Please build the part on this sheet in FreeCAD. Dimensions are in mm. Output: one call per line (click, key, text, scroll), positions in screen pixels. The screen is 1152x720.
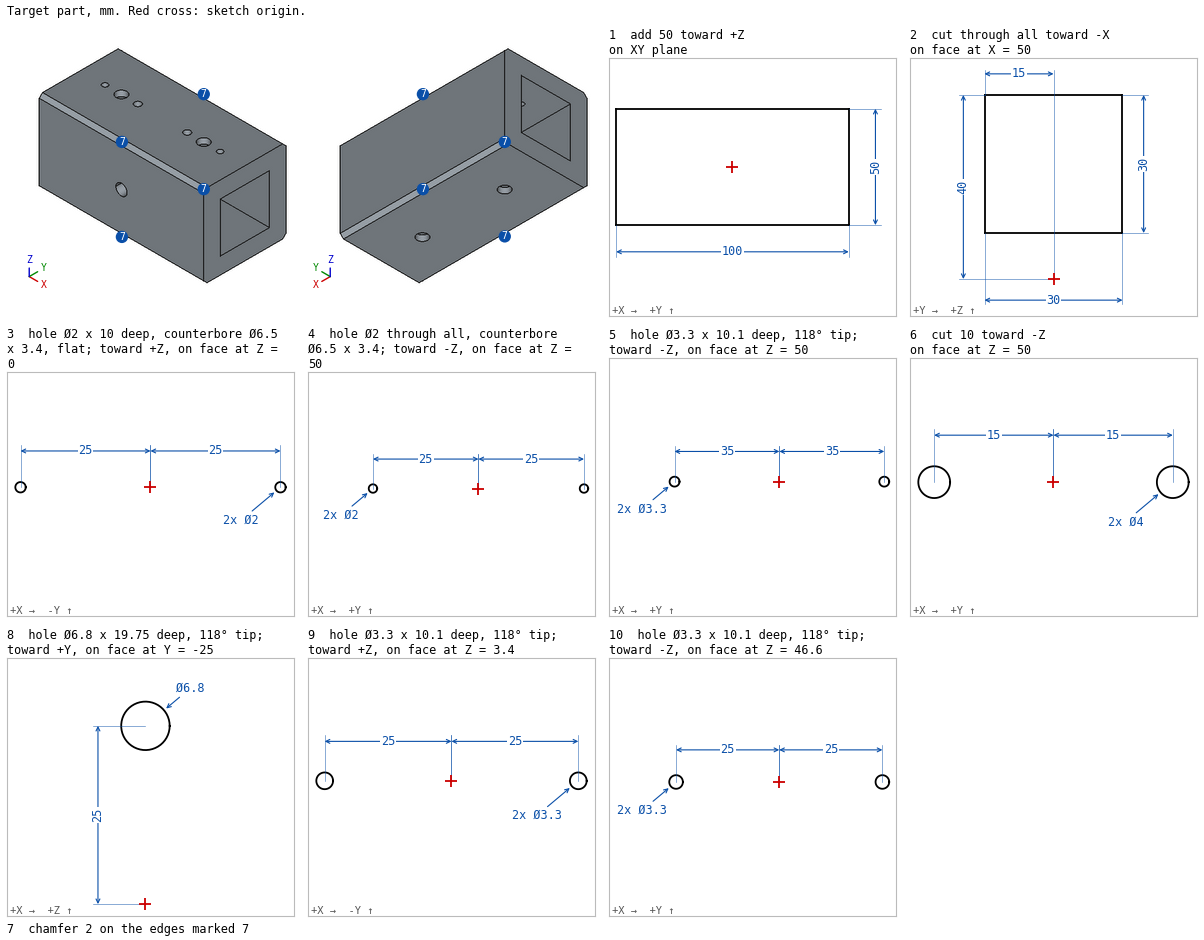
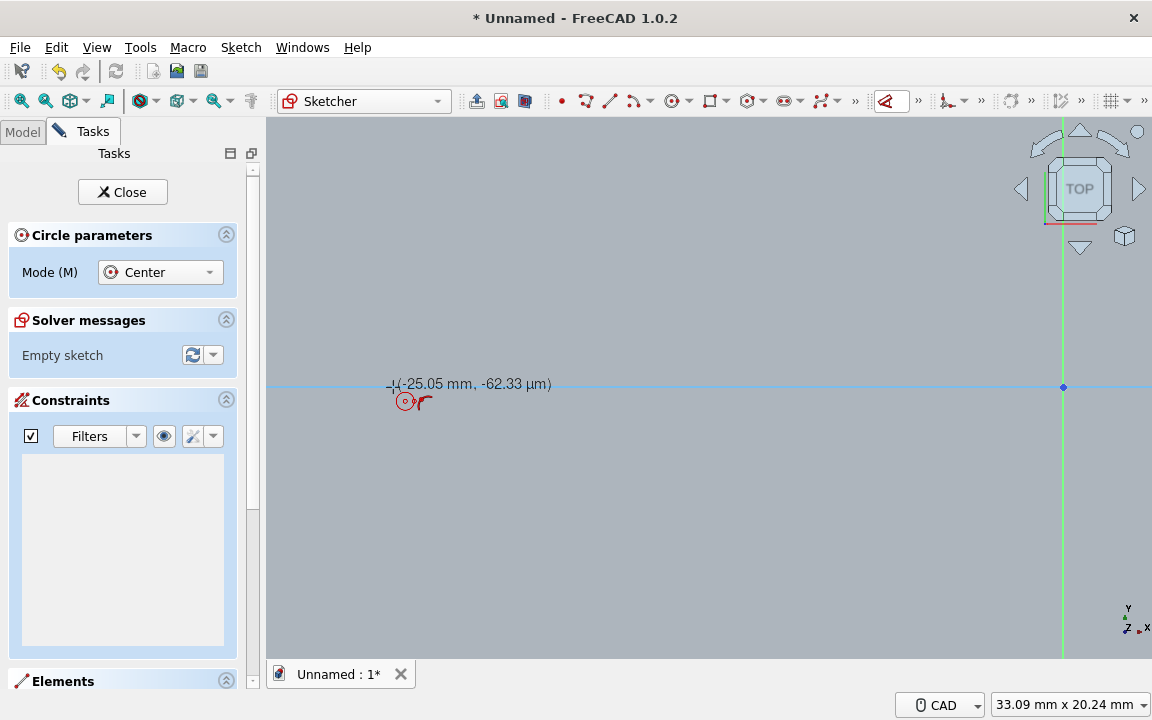
click(394, 387)
move(413, 368)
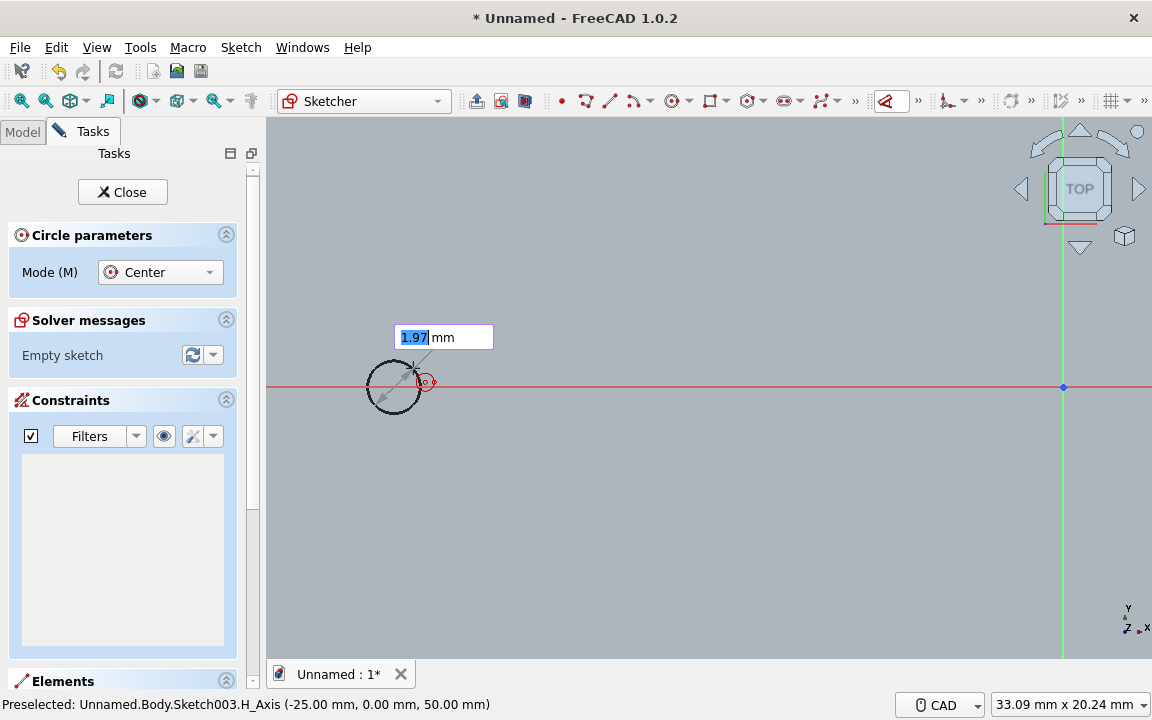
text(2)
key(Return)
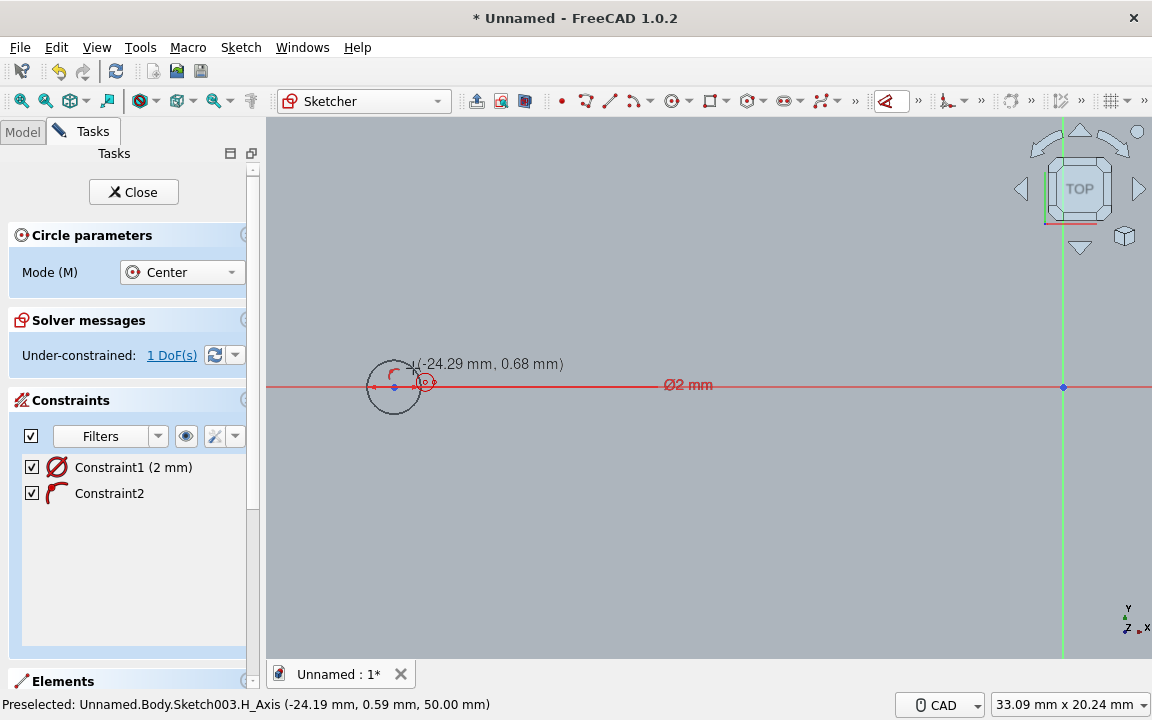
scroll(394, 388, down, 5)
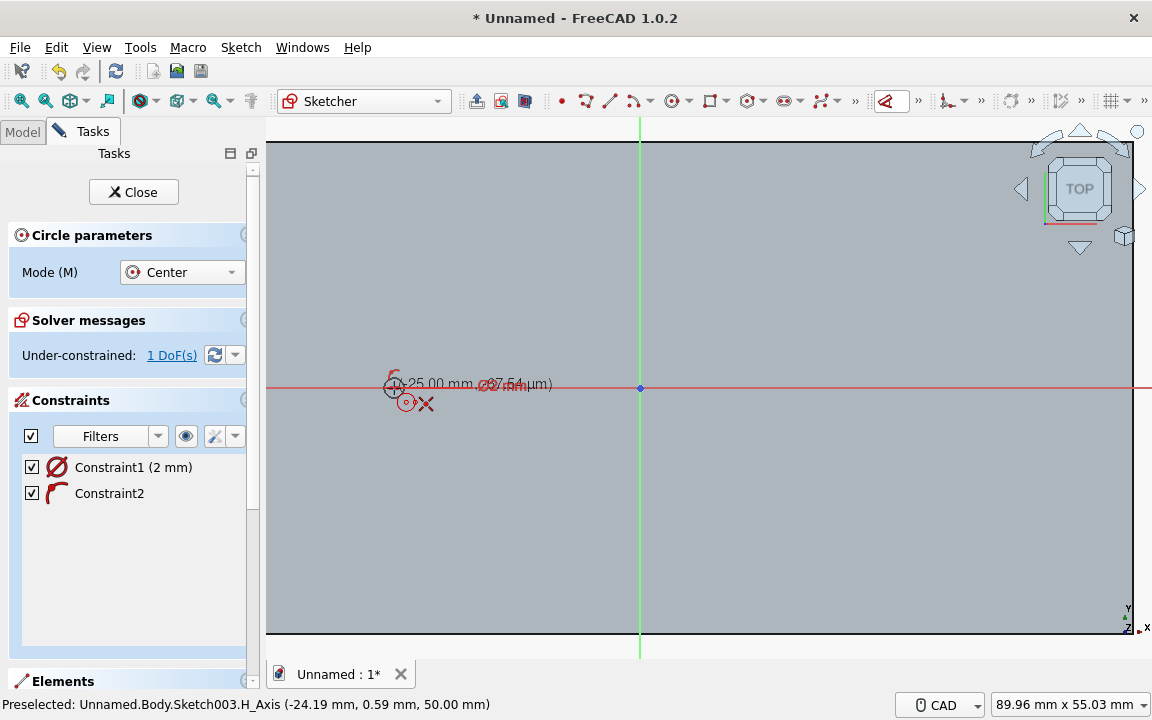
scroll(887, 388, up, 5)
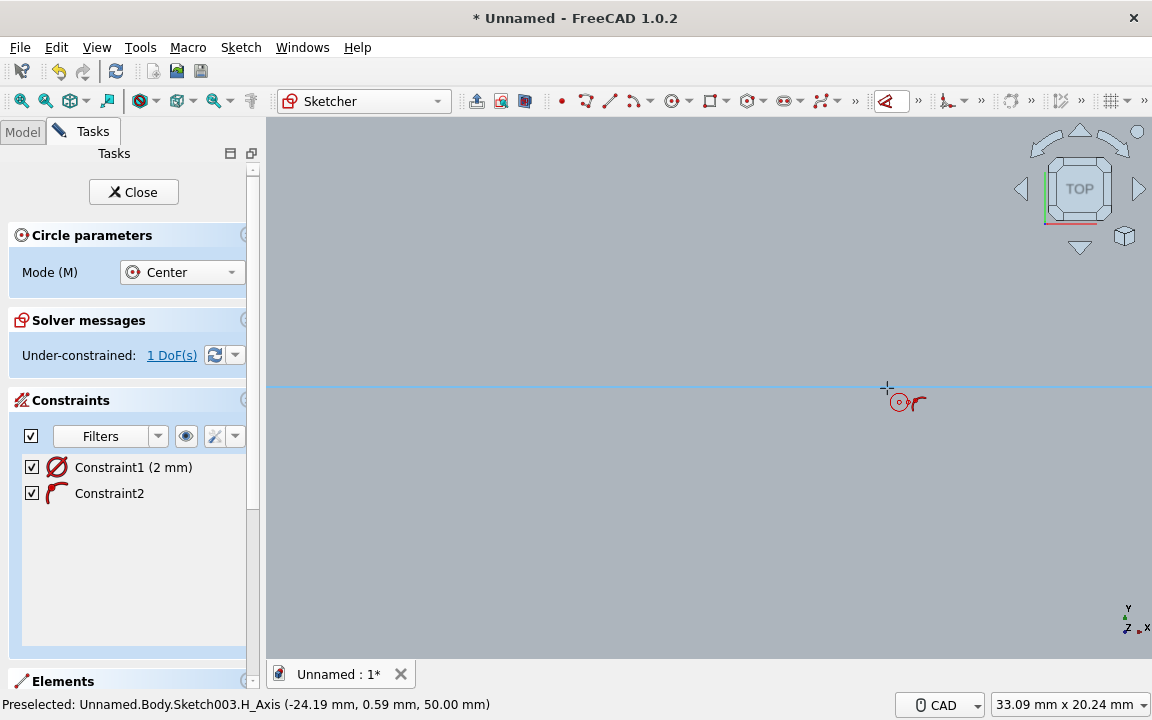
click(885, 387)
move(903, 368)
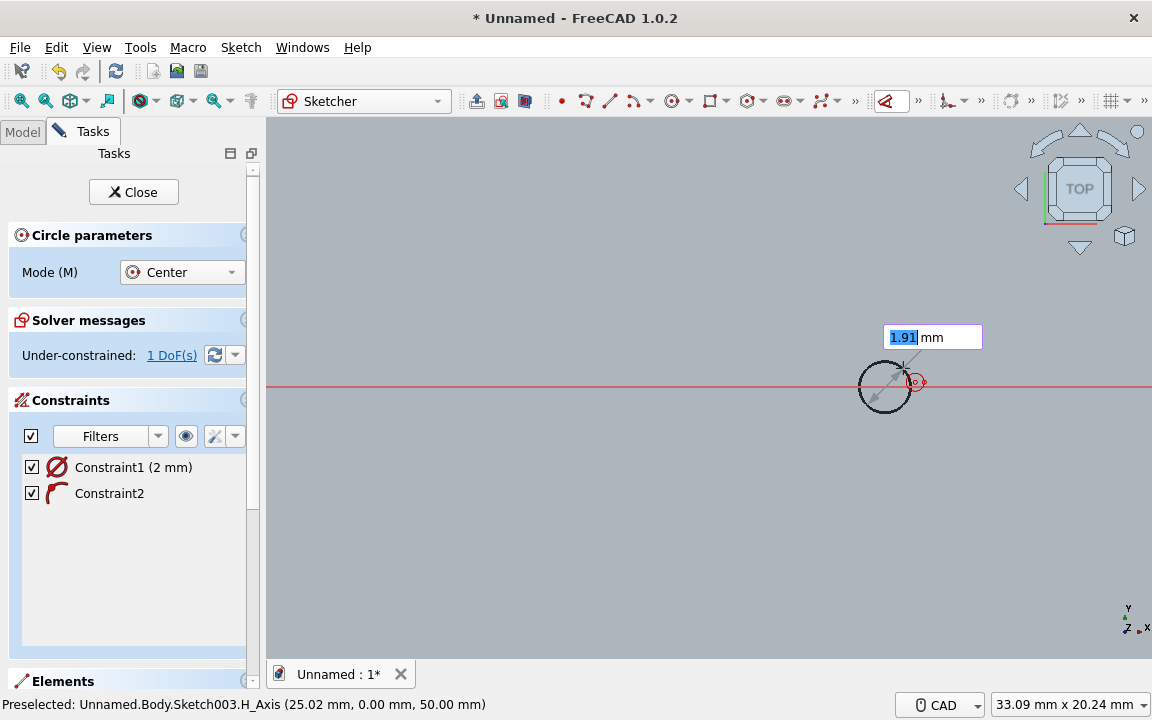
text(2)
key(Return)
key(Escape)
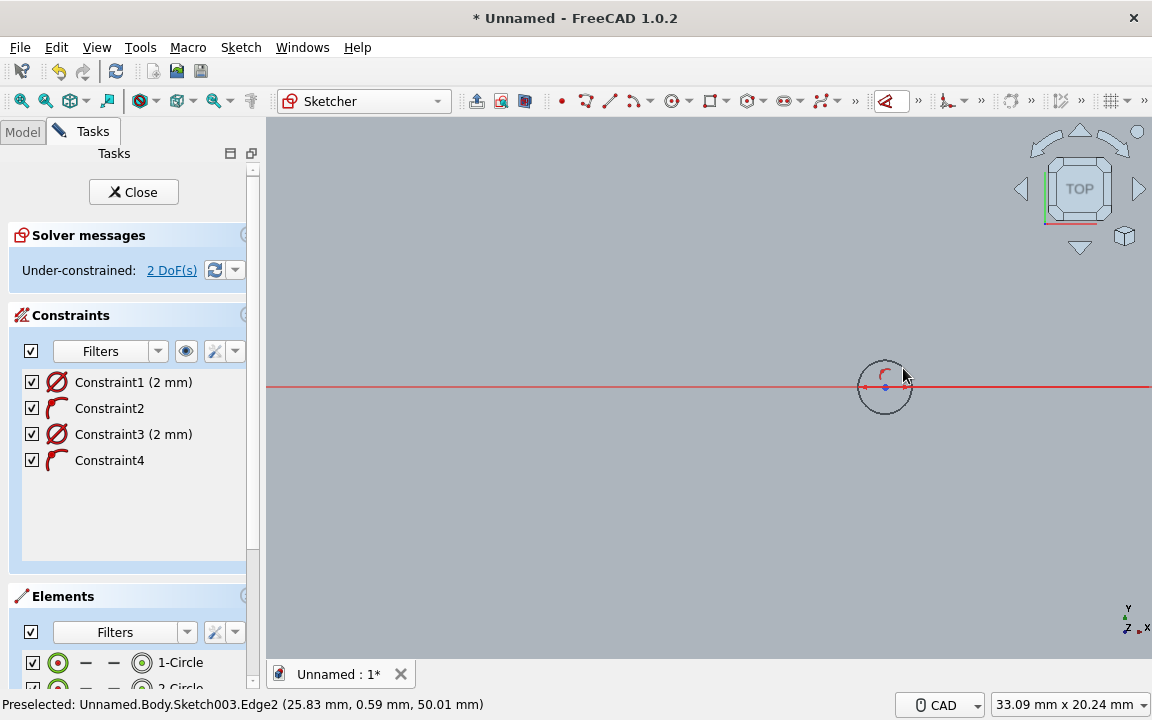
scroll(888, 388, down, 5)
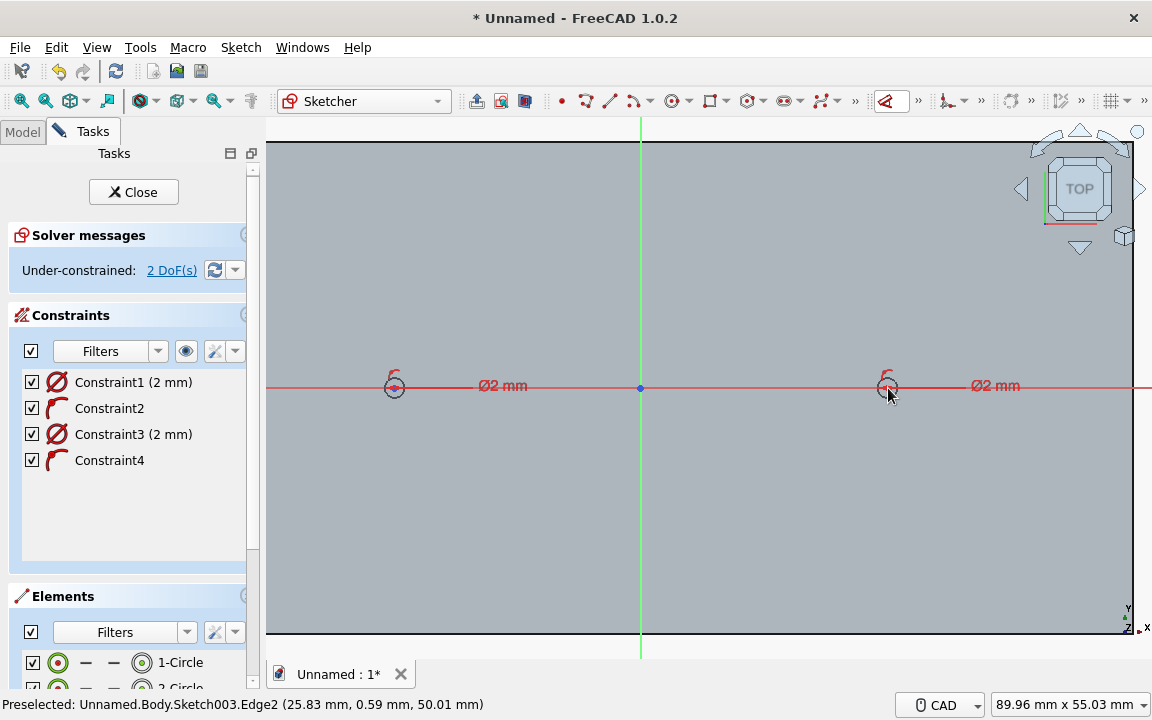
click(395, 388)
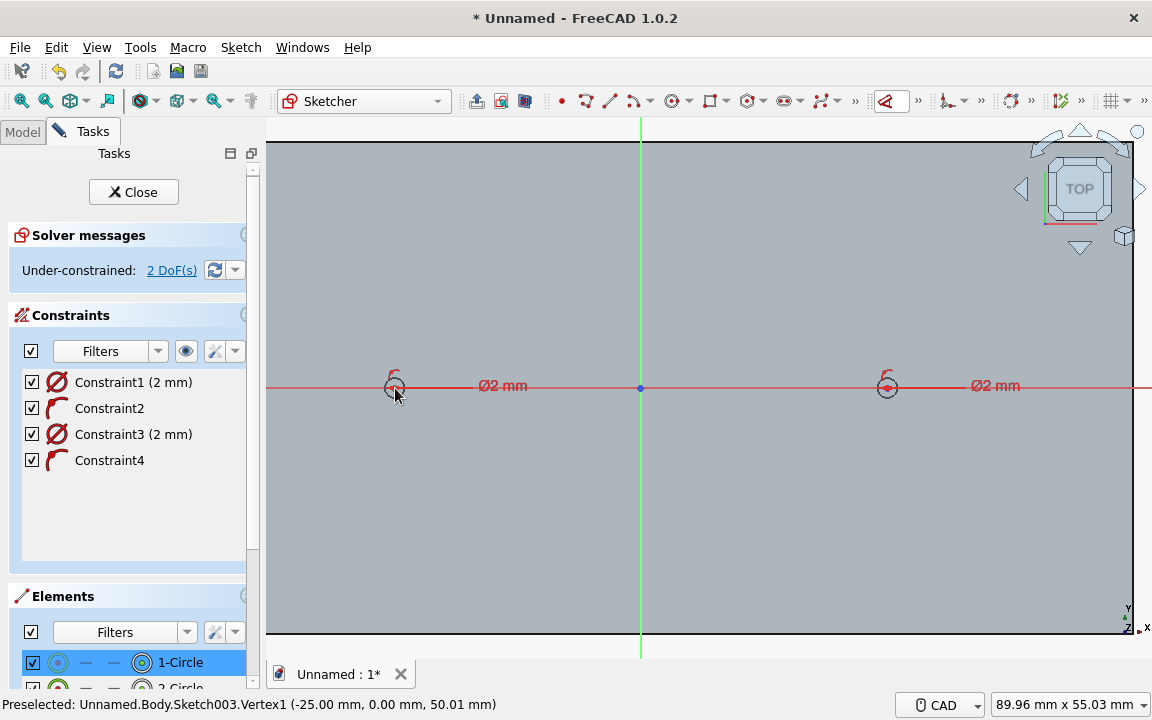
key(l)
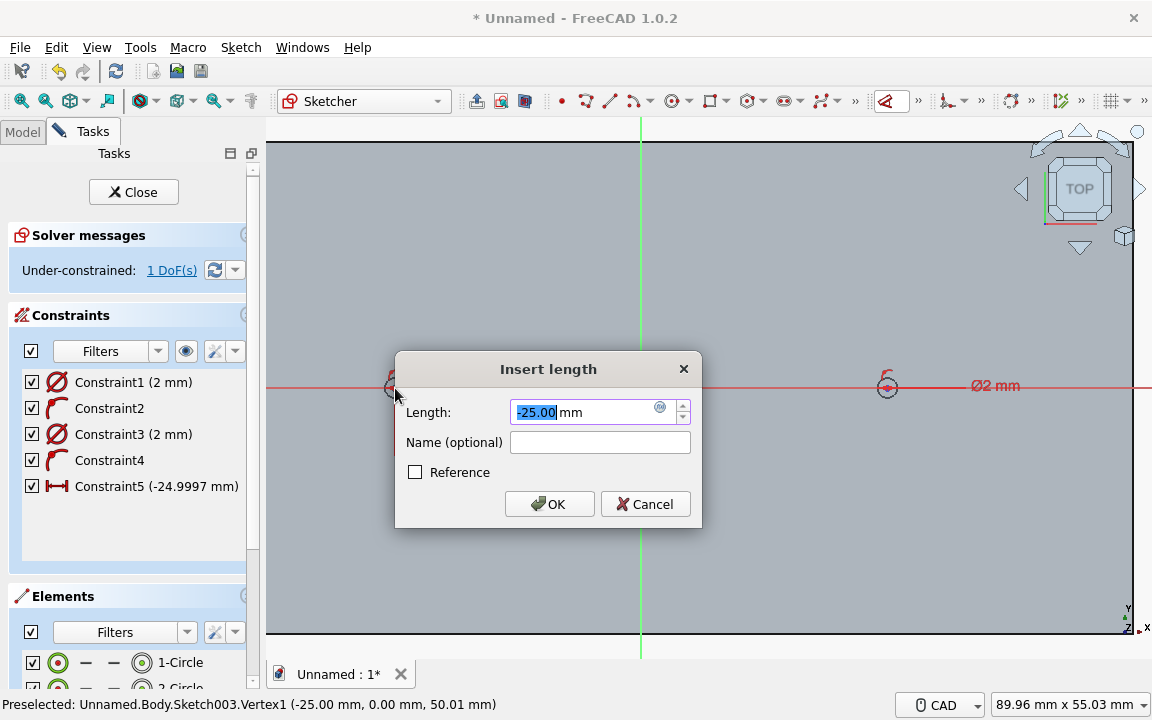
text(-25)
key(Return)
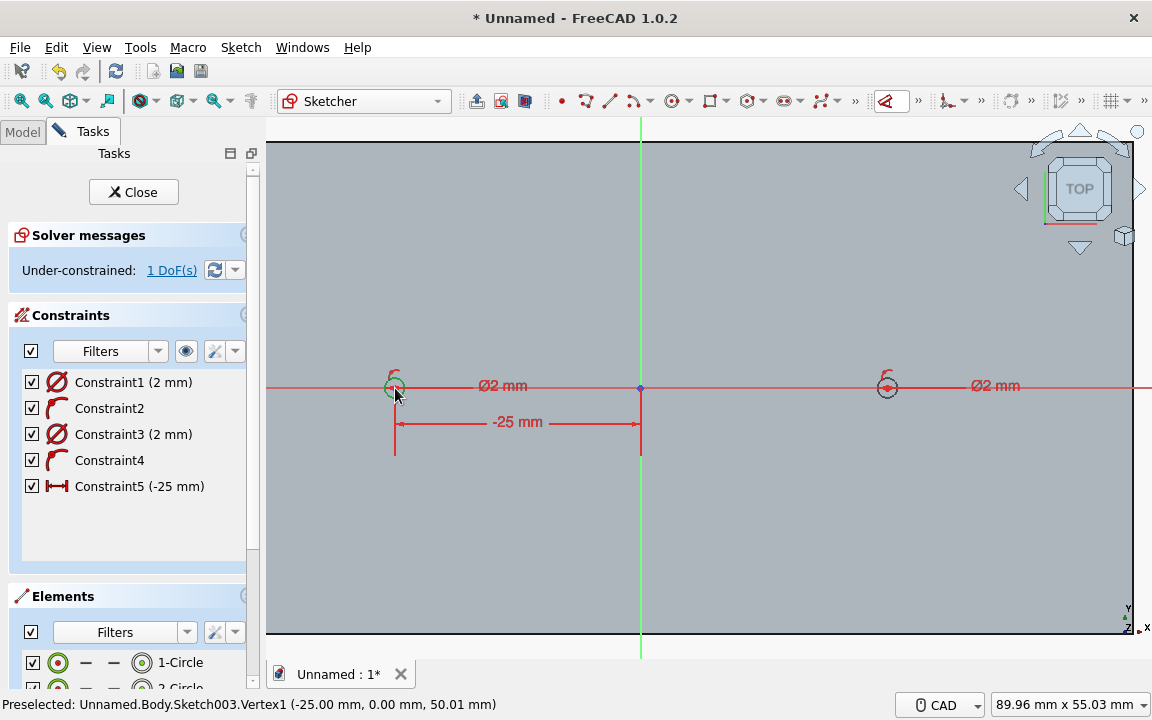
click(887, 388)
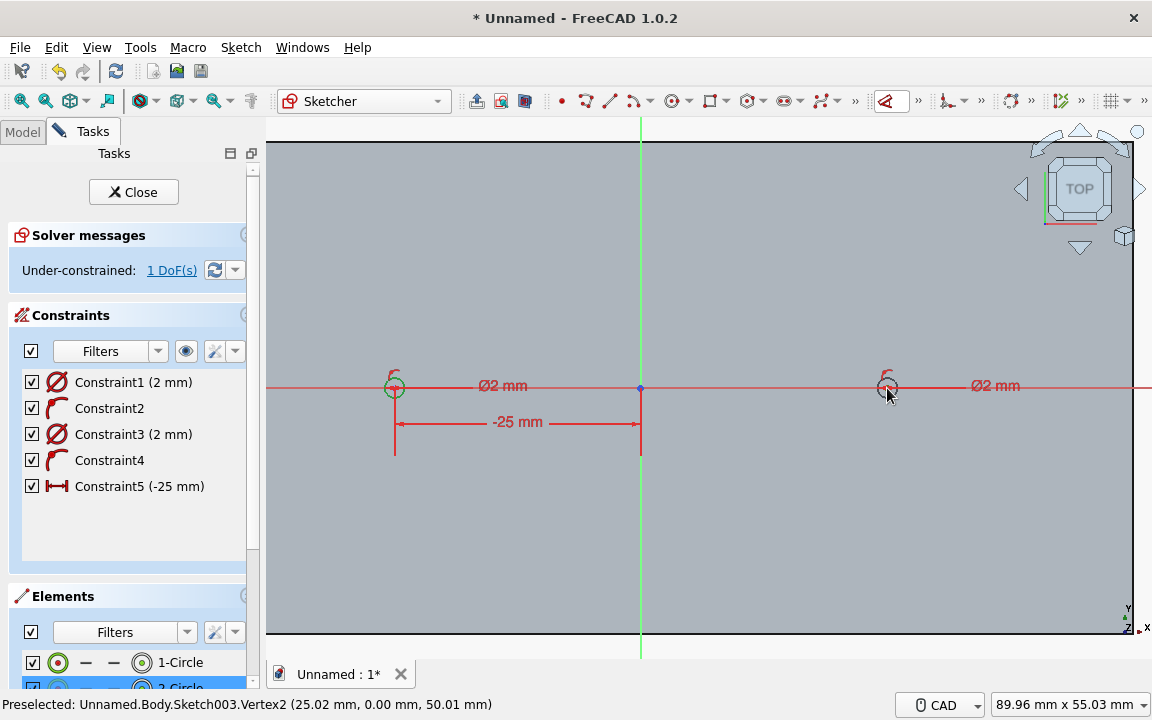
click(904, 102)